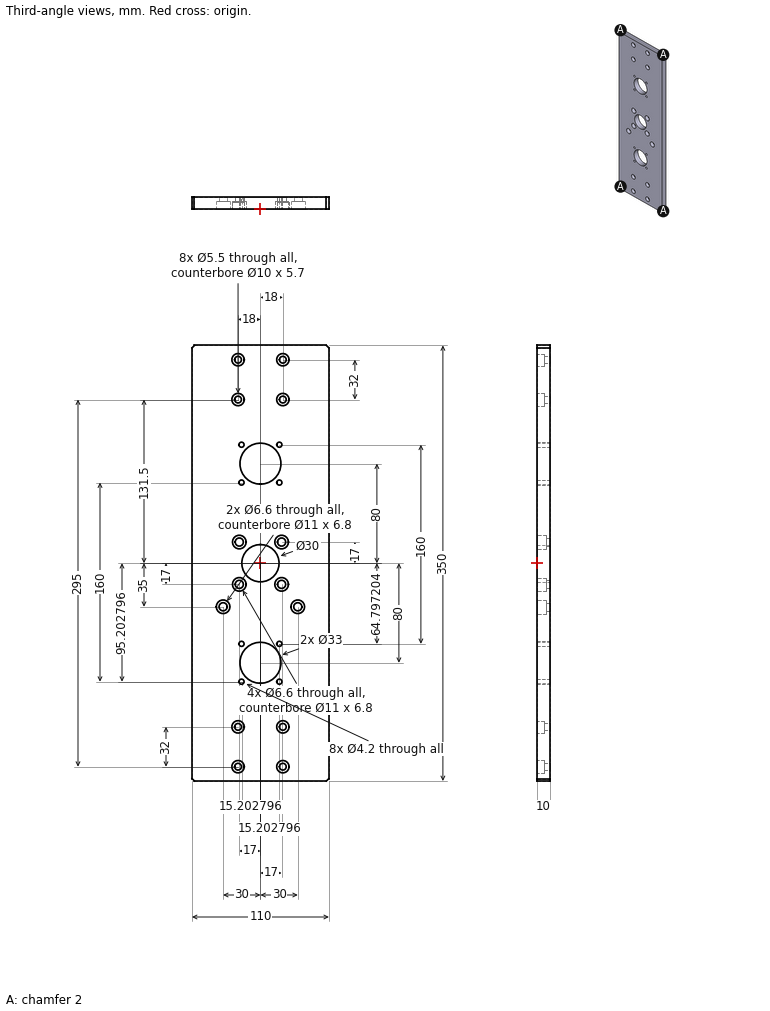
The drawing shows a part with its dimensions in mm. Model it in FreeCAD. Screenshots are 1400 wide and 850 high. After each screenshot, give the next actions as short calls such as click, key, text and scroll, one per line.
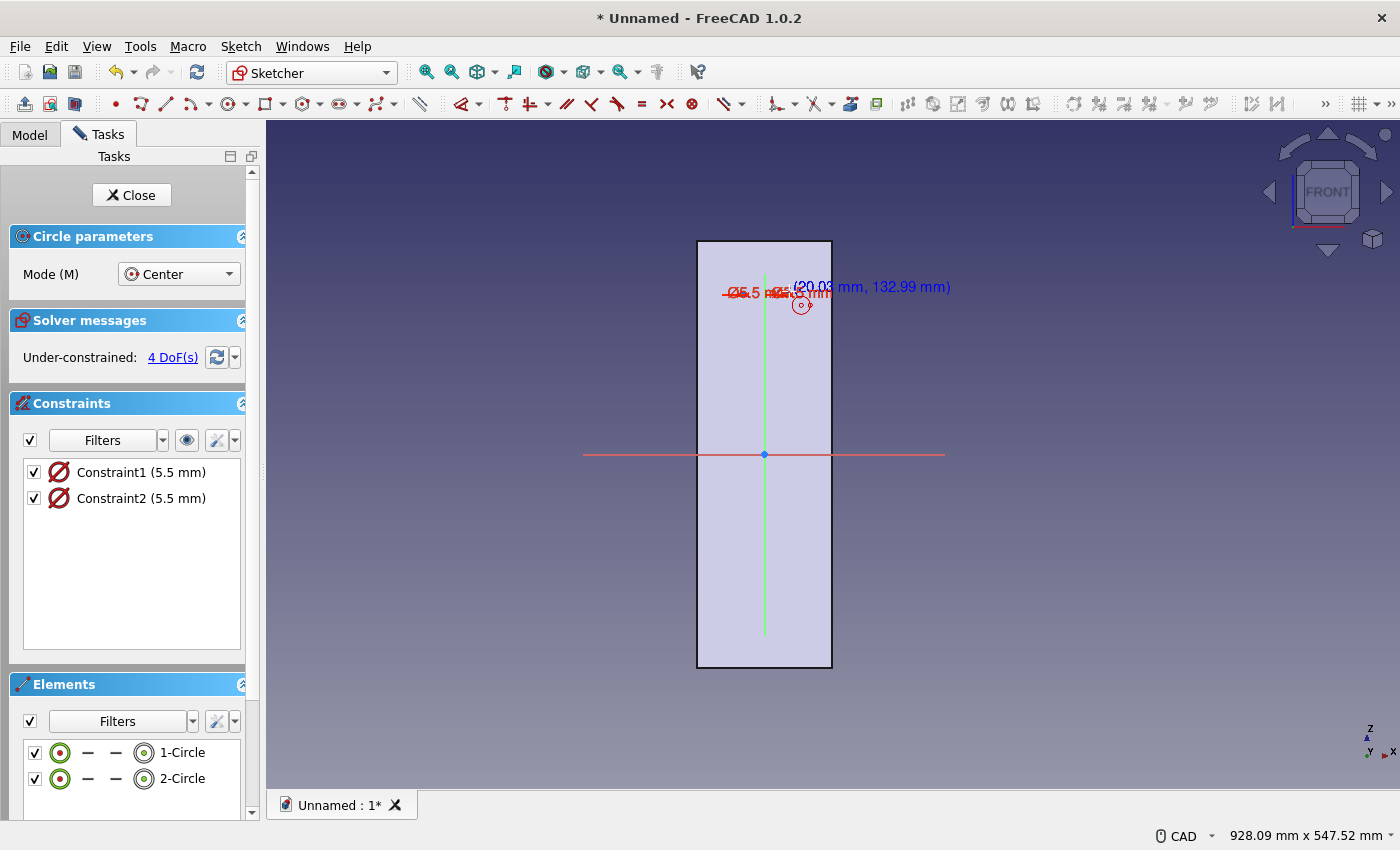
scroll(787, 255, up, 10)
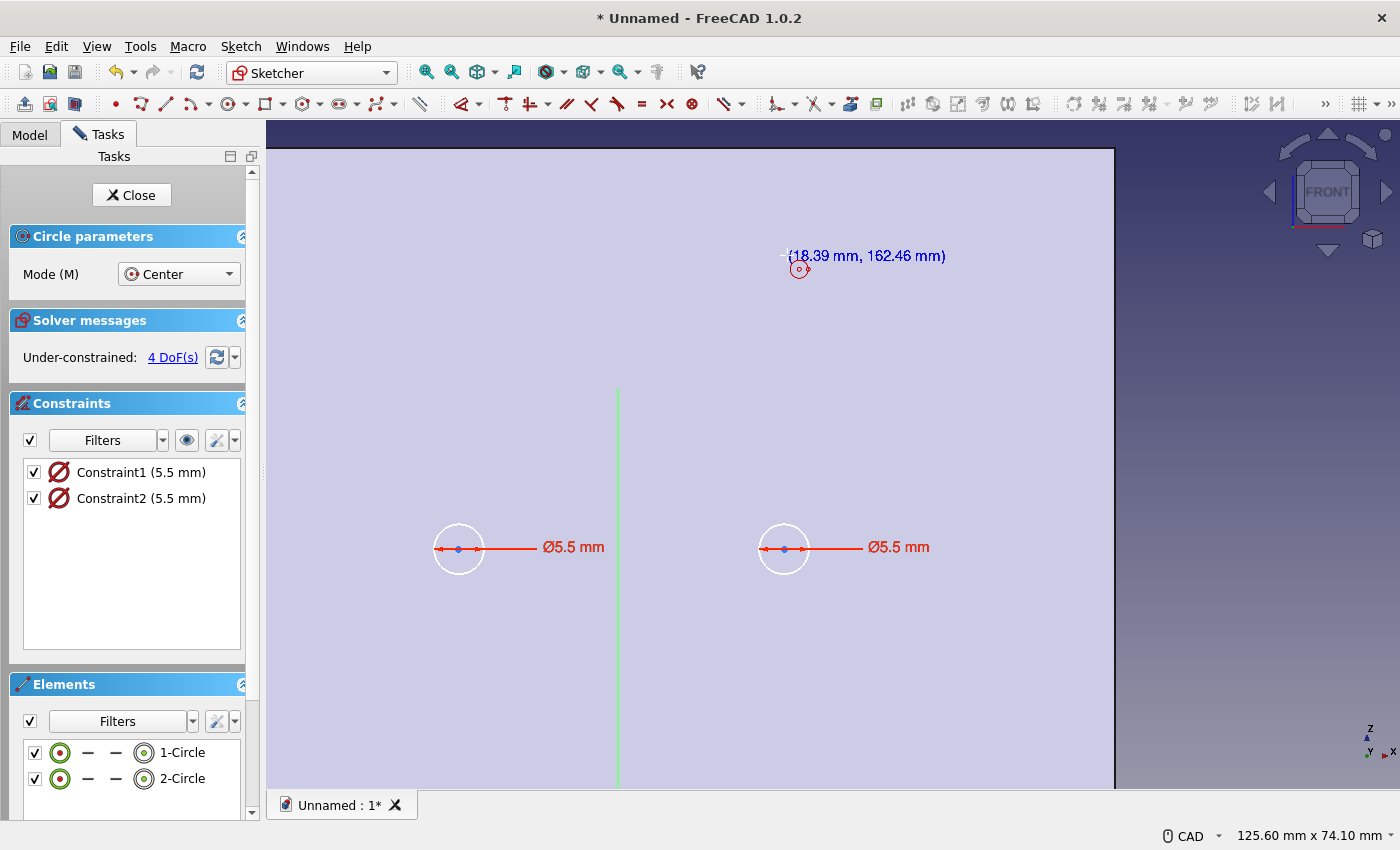
scroll(787, 255, down, 10)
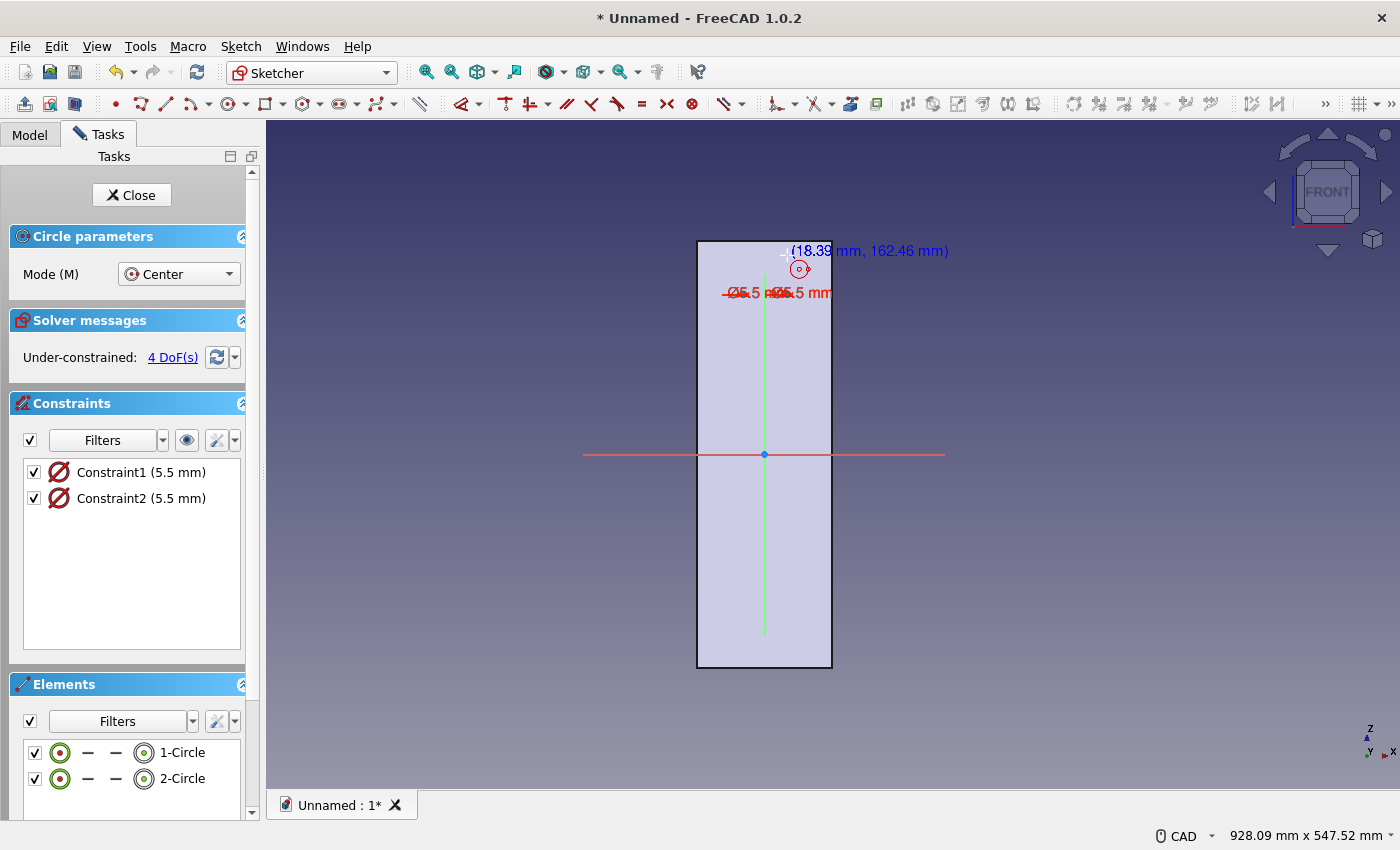
click(787, 255)
move(789, 252)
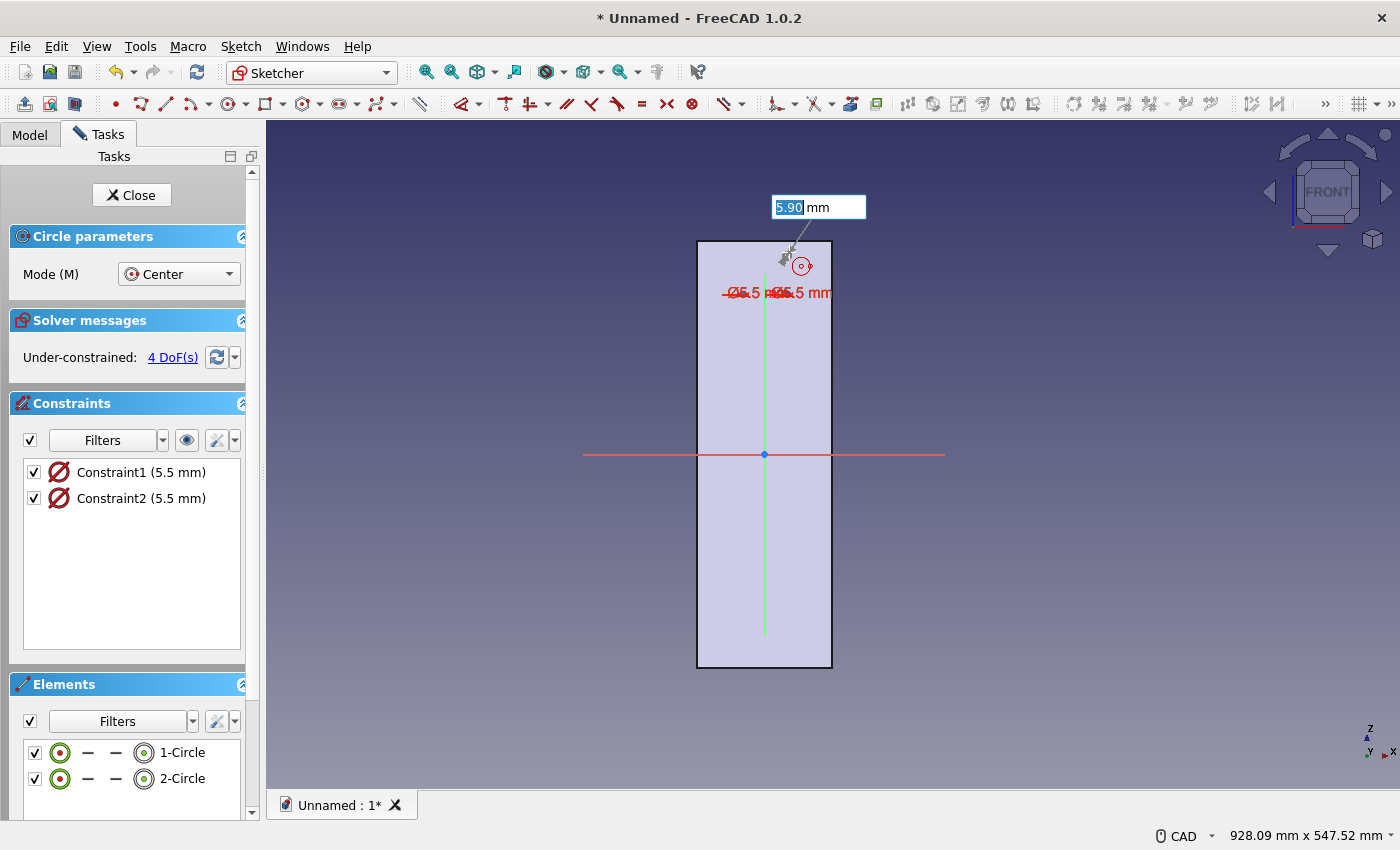
text(5.5)
key(Return)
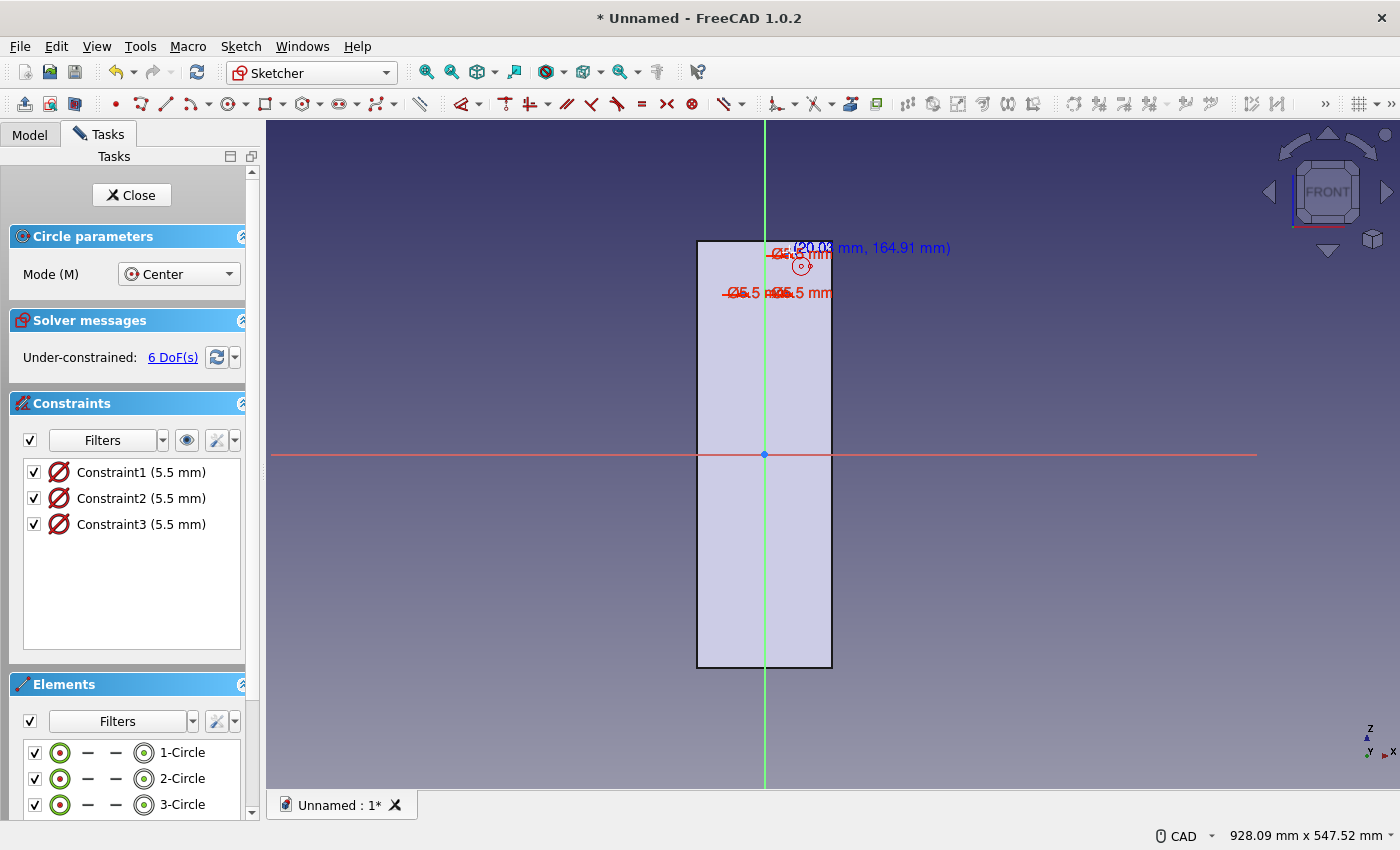
scroll(743, 255, up, 10)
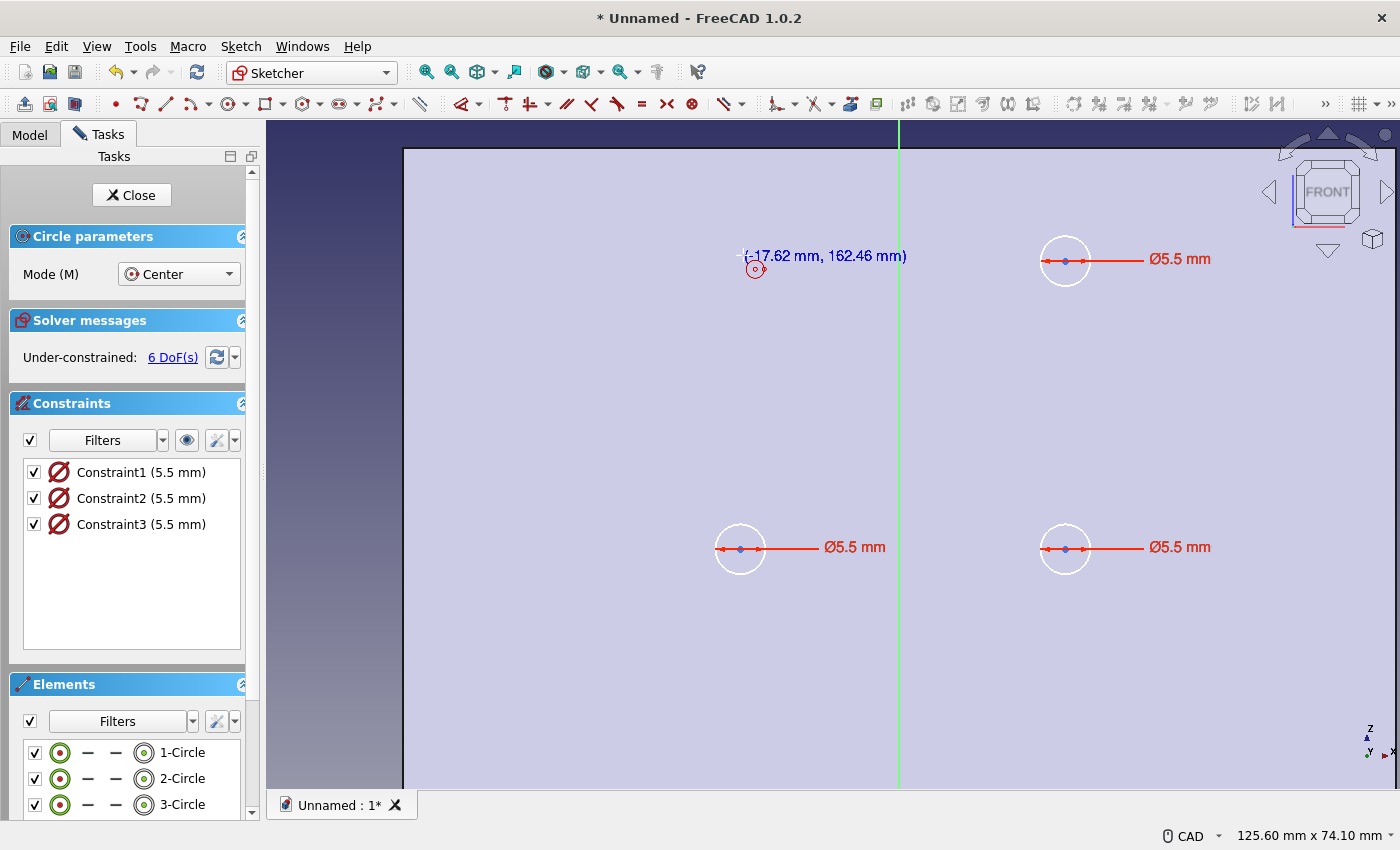
scroll(743, 255, down, 10)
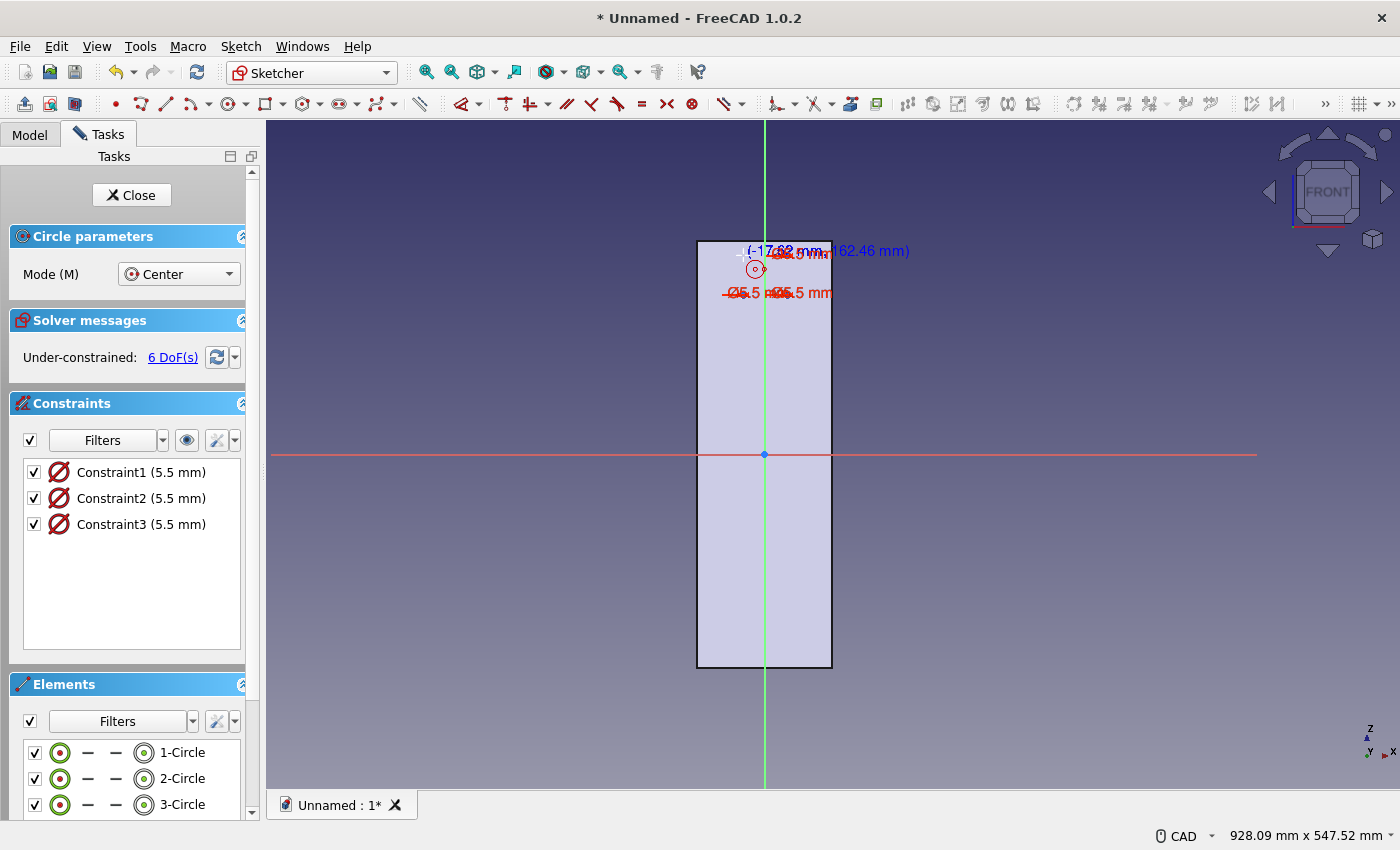
click(743, 255)
move(745, 252)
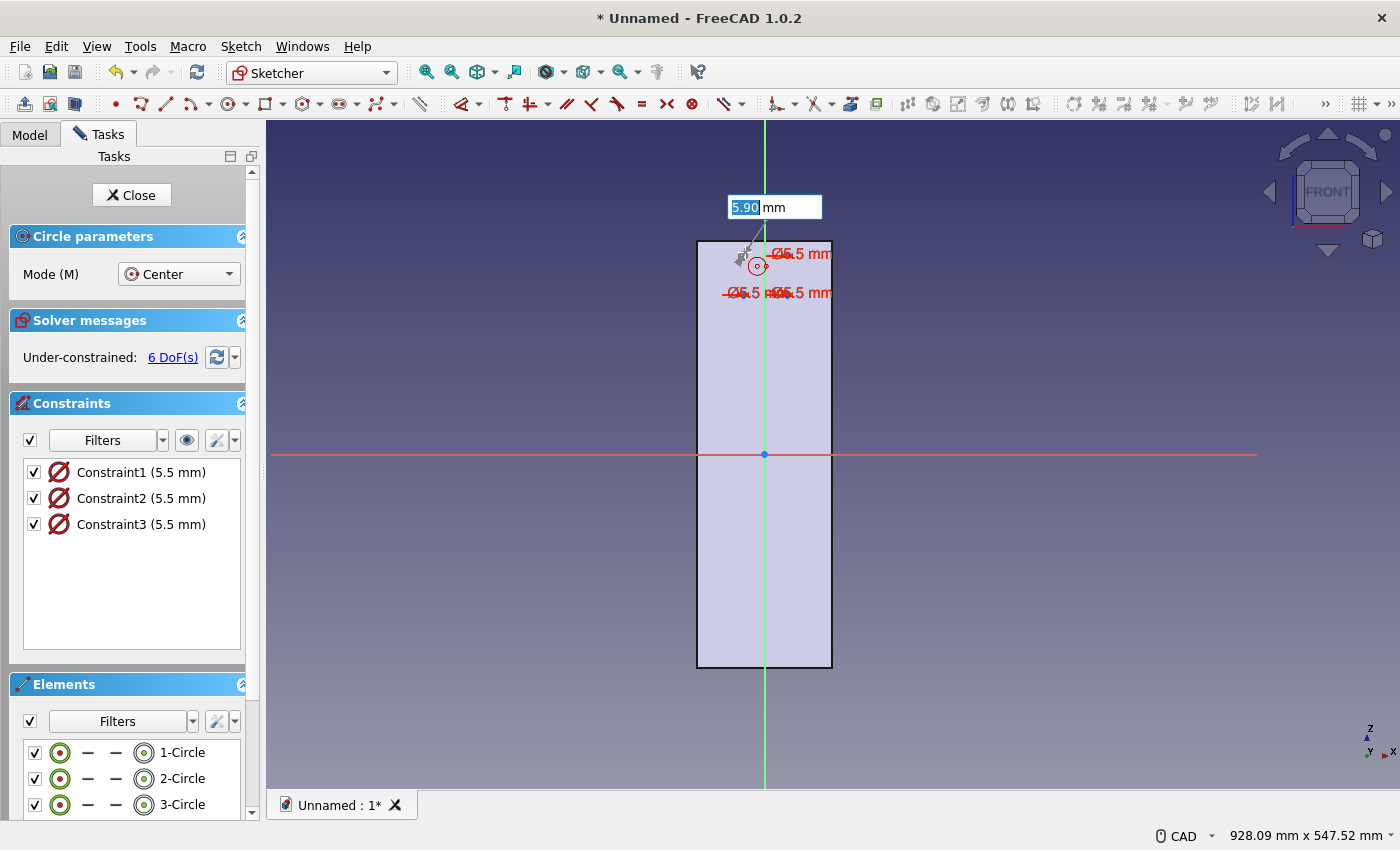
text(5.5)
key(Return)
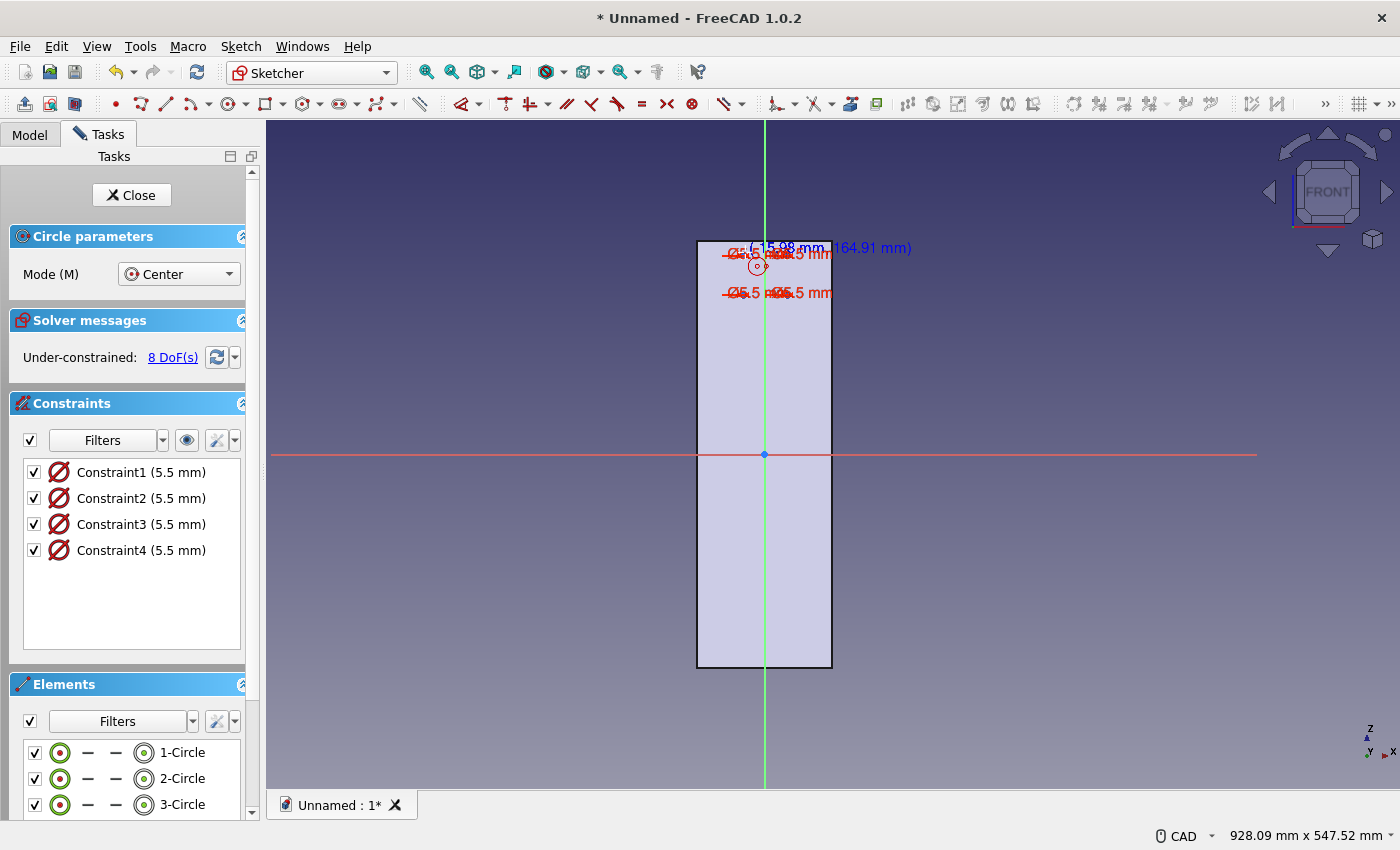
scroll(743, 654, up, 10)